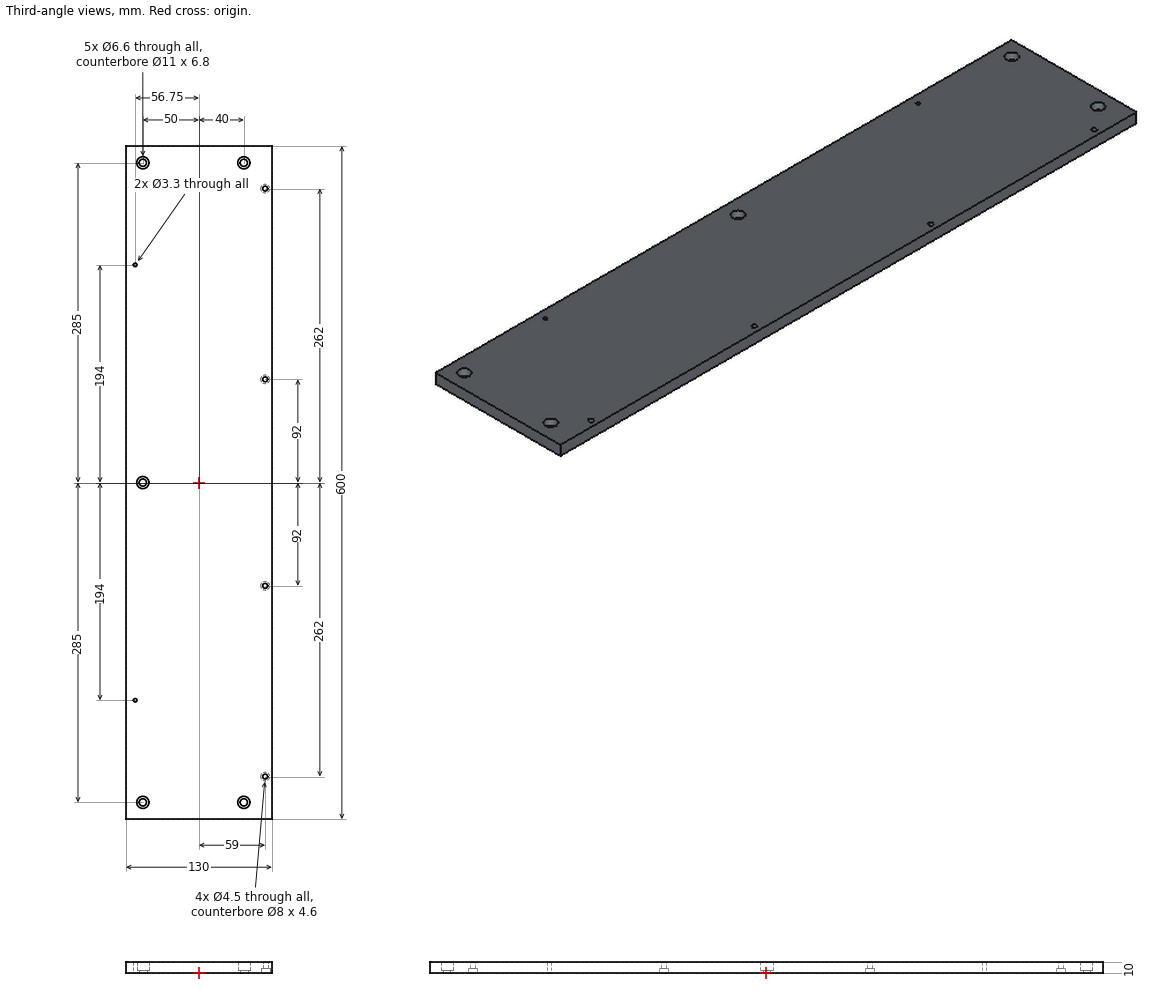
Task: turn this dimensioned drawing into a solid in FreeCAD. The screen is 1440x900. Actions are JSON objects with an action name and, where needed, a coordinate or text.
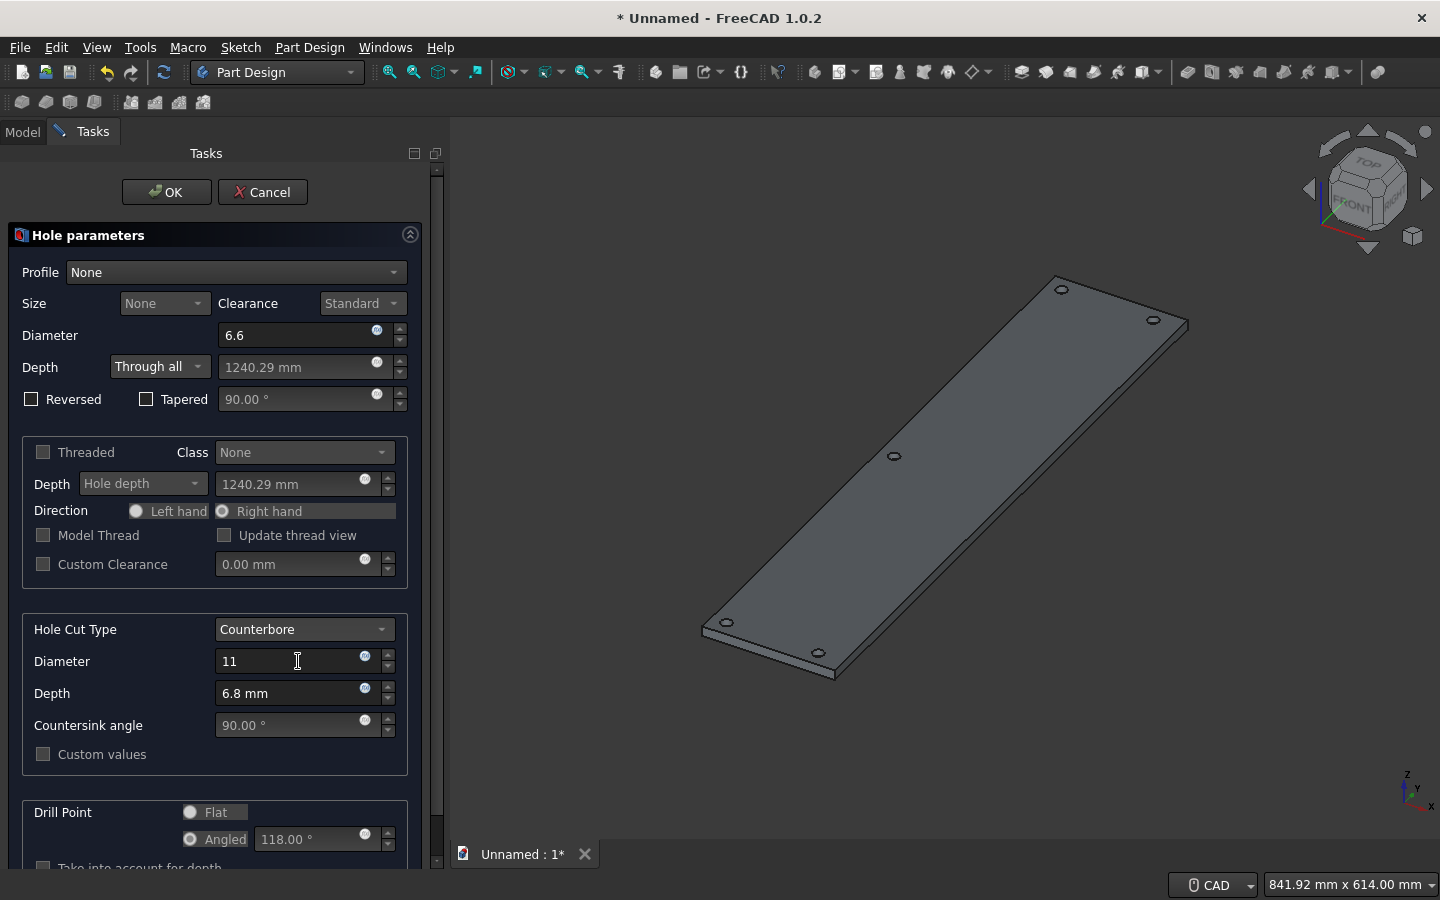
{"action": "left_click", "coordinate": [167, 192]}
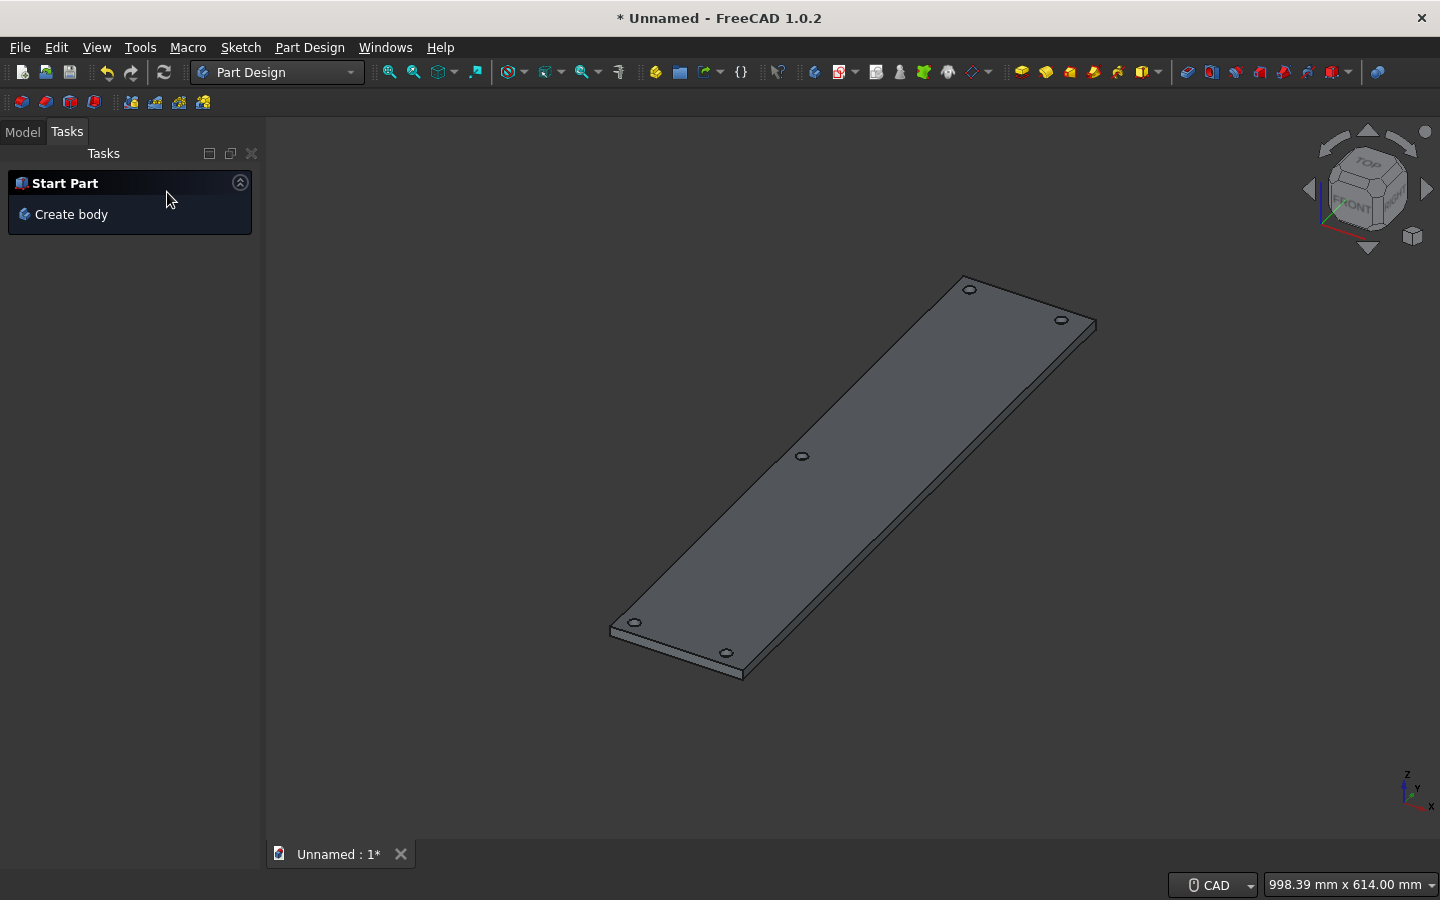
{"action": "left_click", "coordinate": [954, 372]}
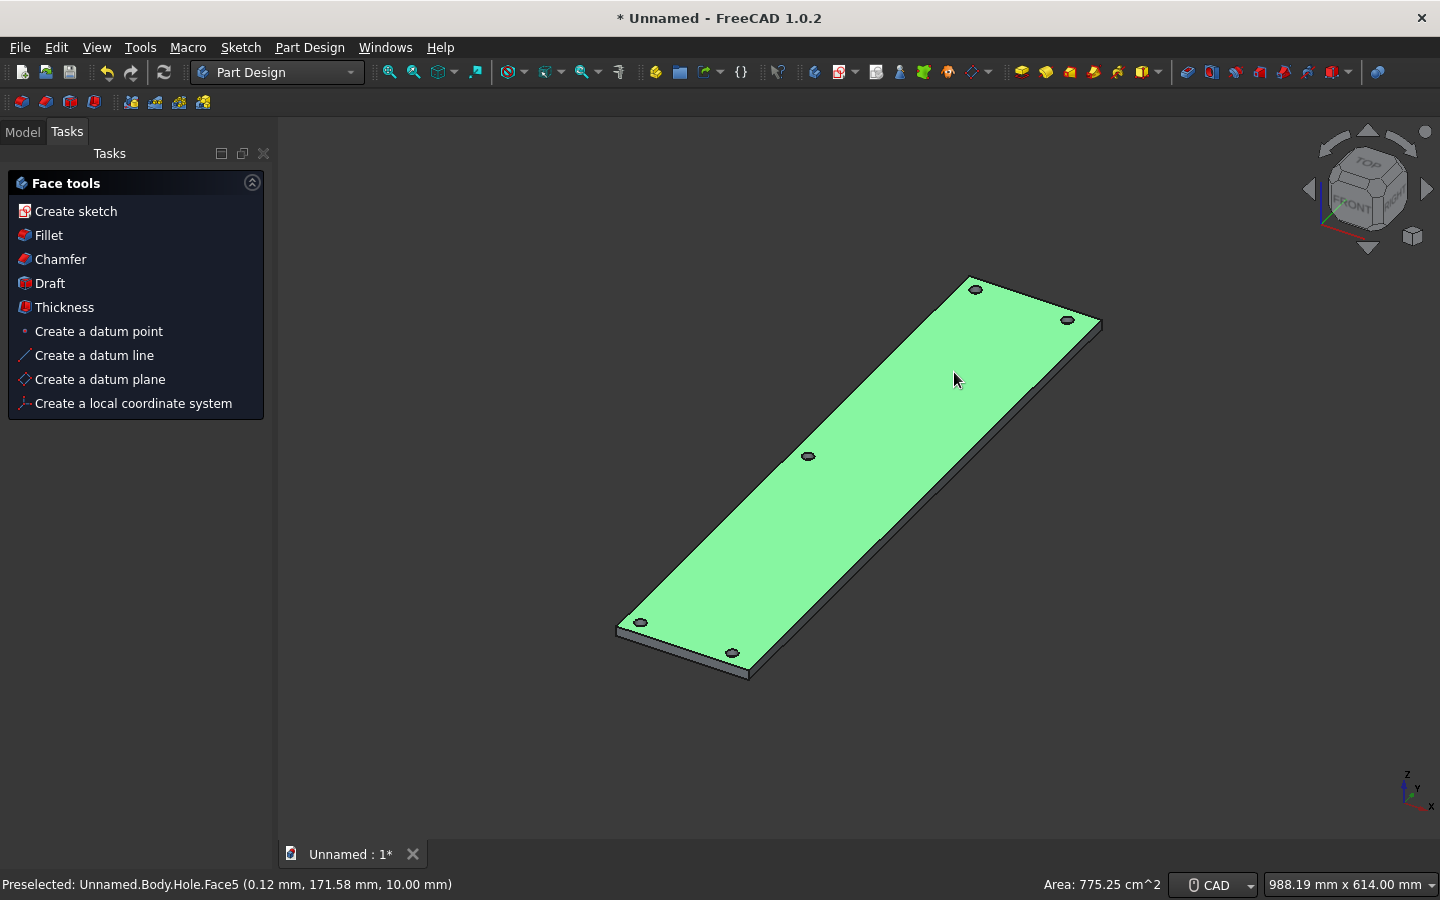
{"action": "left_click", "coordinate": [840, 72]}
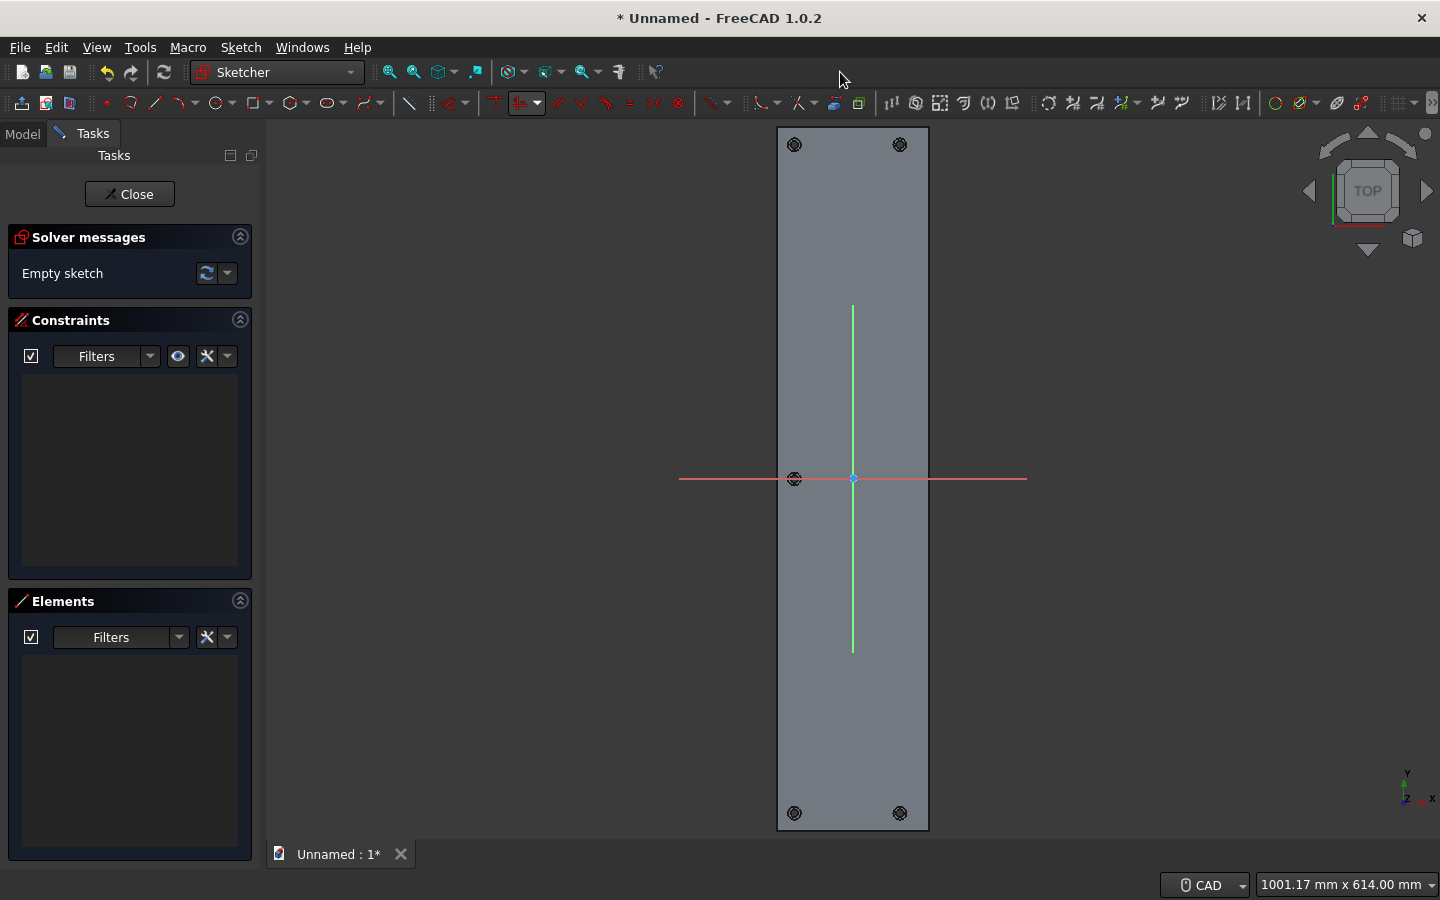
{"action": "key", "text": "g c"}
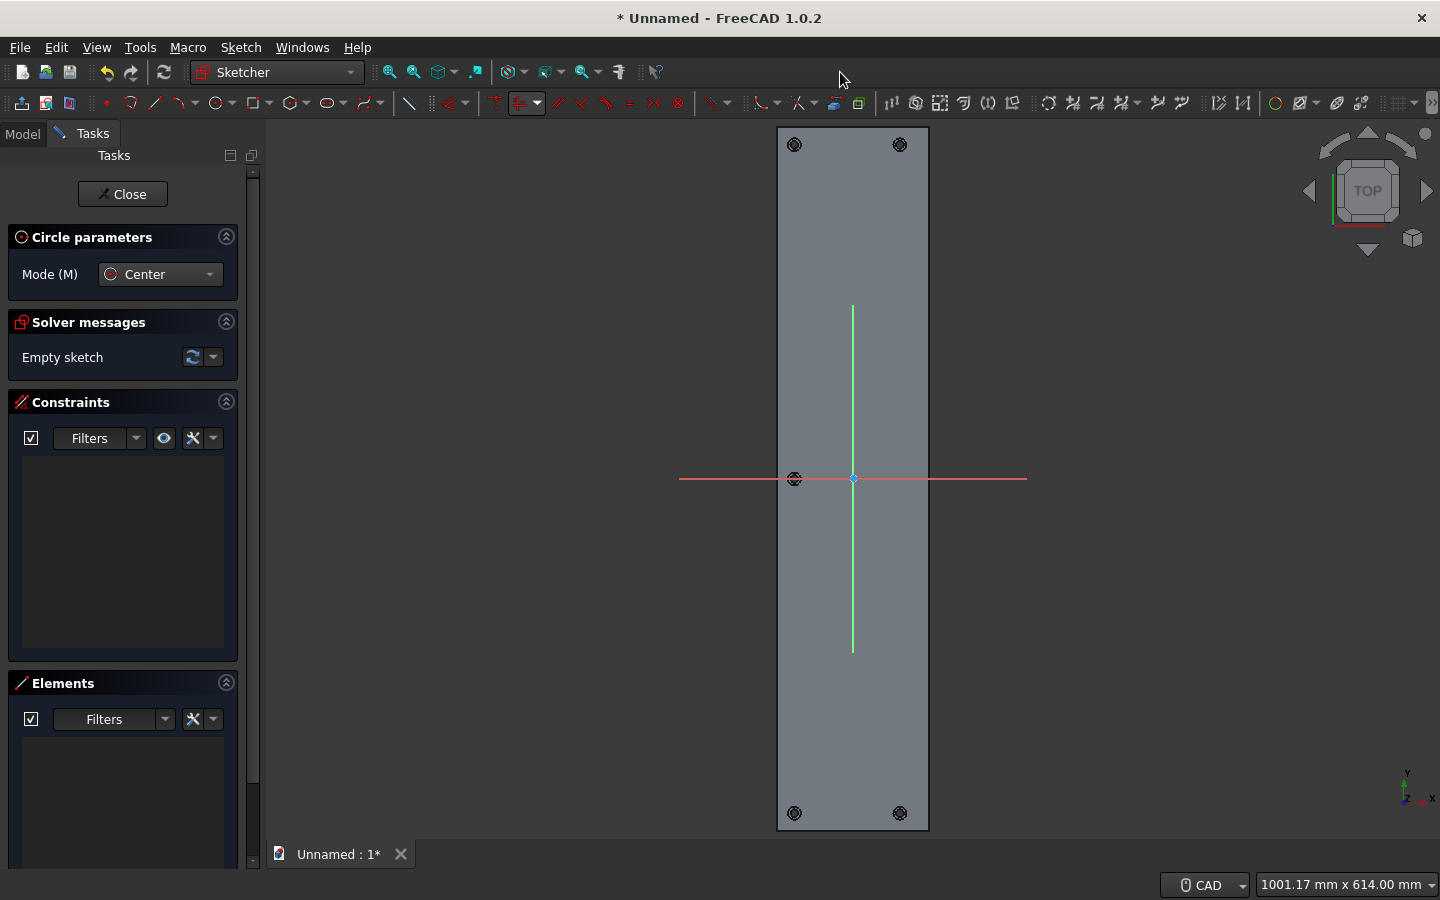
{"action": "scroll", "coordinate": [786, 252], "scroll_direction": "up", "scroll_amount": 13}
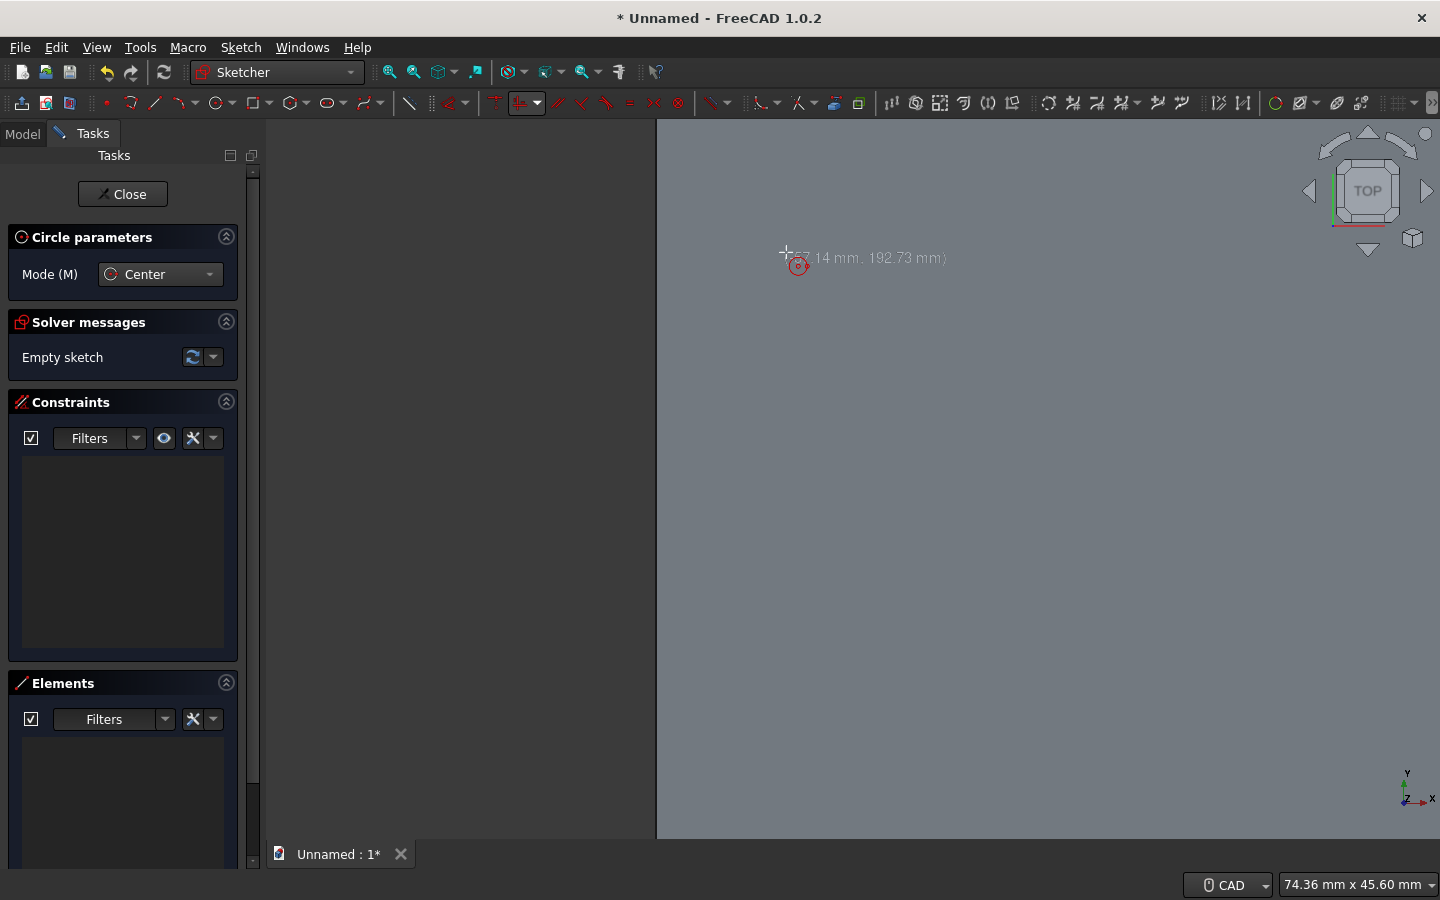
{"action": "scroll", "coordinate": [749, 252], "scroll_direction": "down", "scroll_amount": 13}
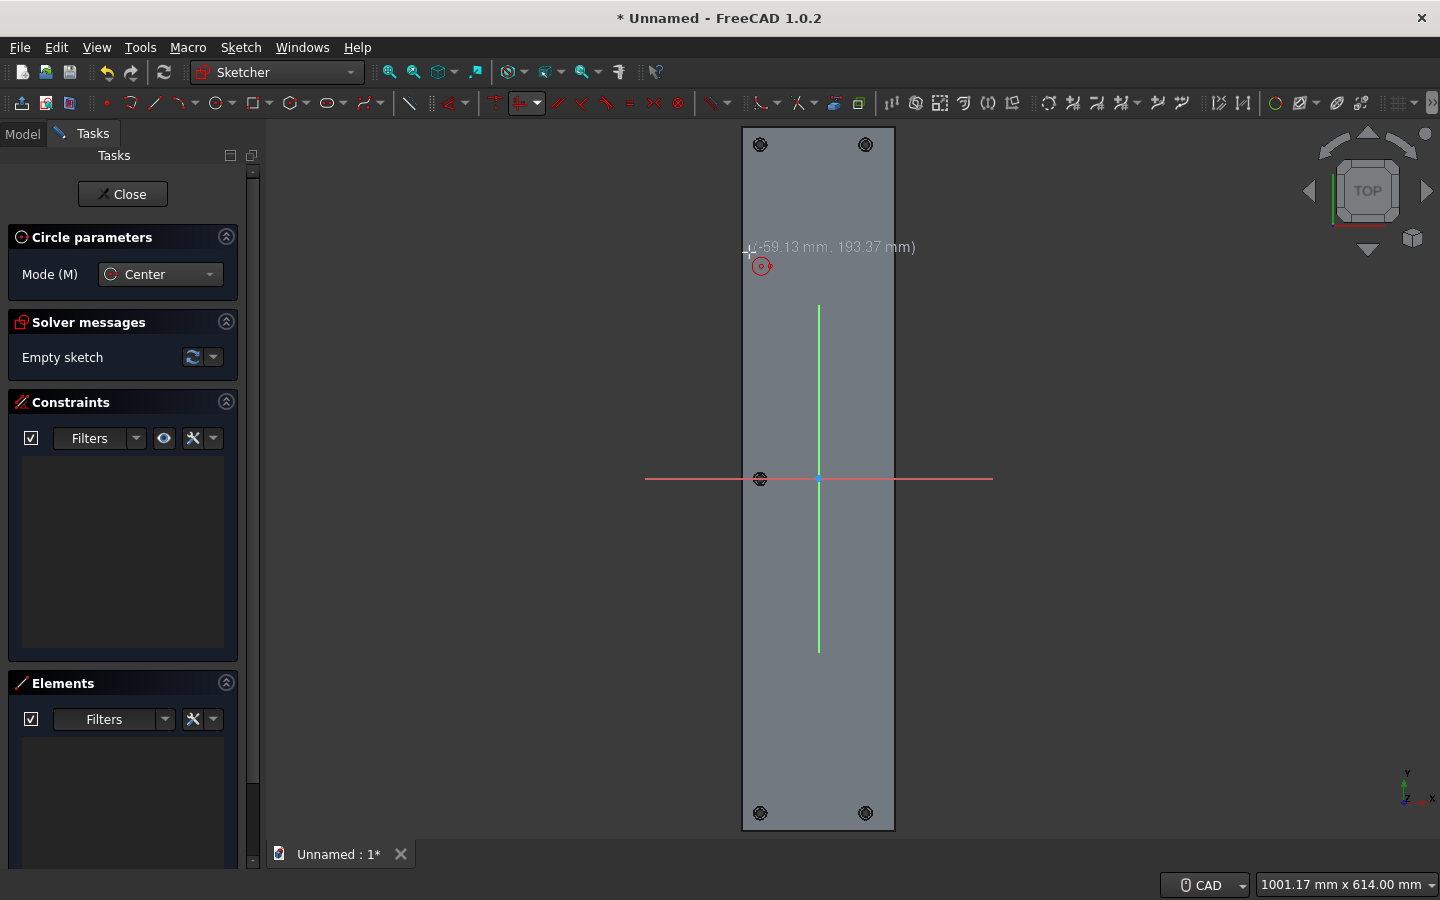
{"action": "left_click", "coordinate": [752, 252]}
{"action": "mouse_move", "coordinate": [754, 250]}